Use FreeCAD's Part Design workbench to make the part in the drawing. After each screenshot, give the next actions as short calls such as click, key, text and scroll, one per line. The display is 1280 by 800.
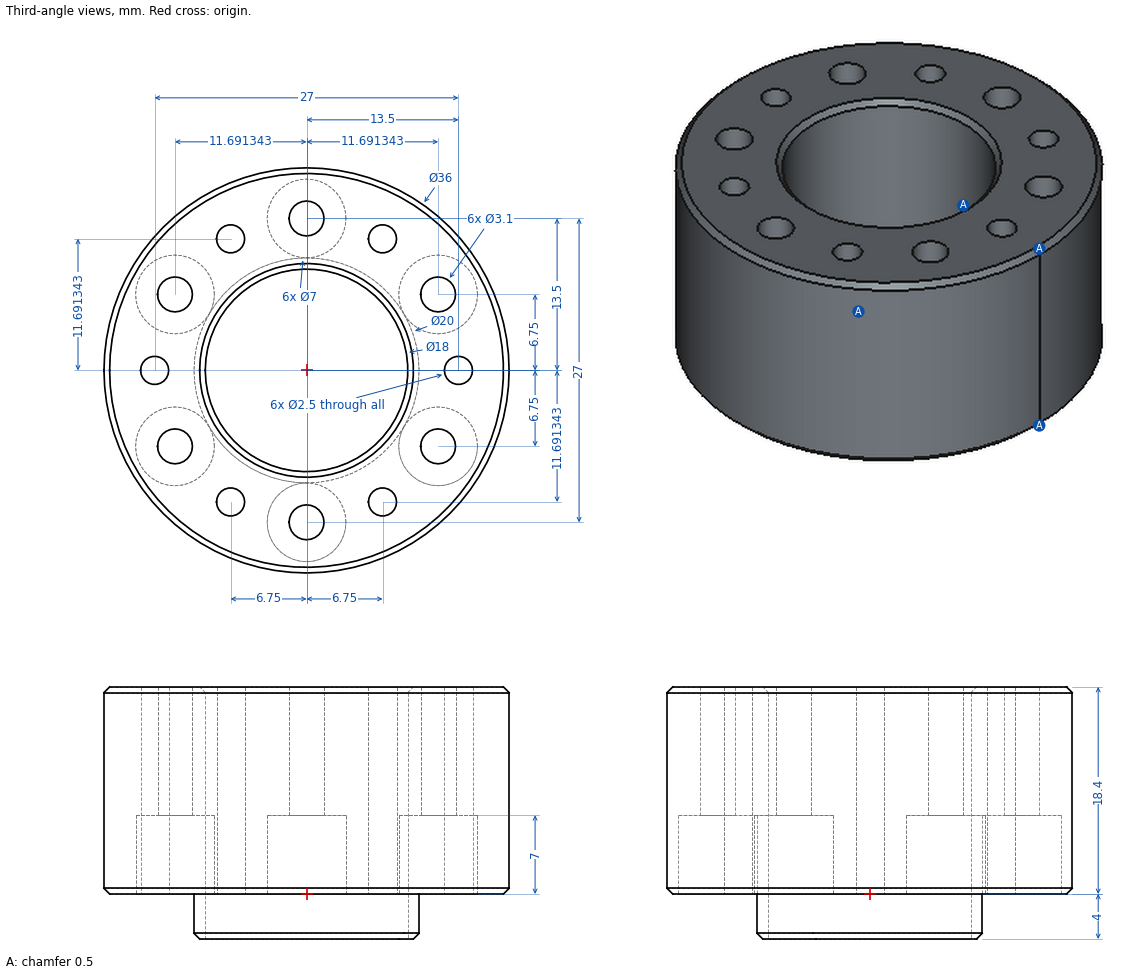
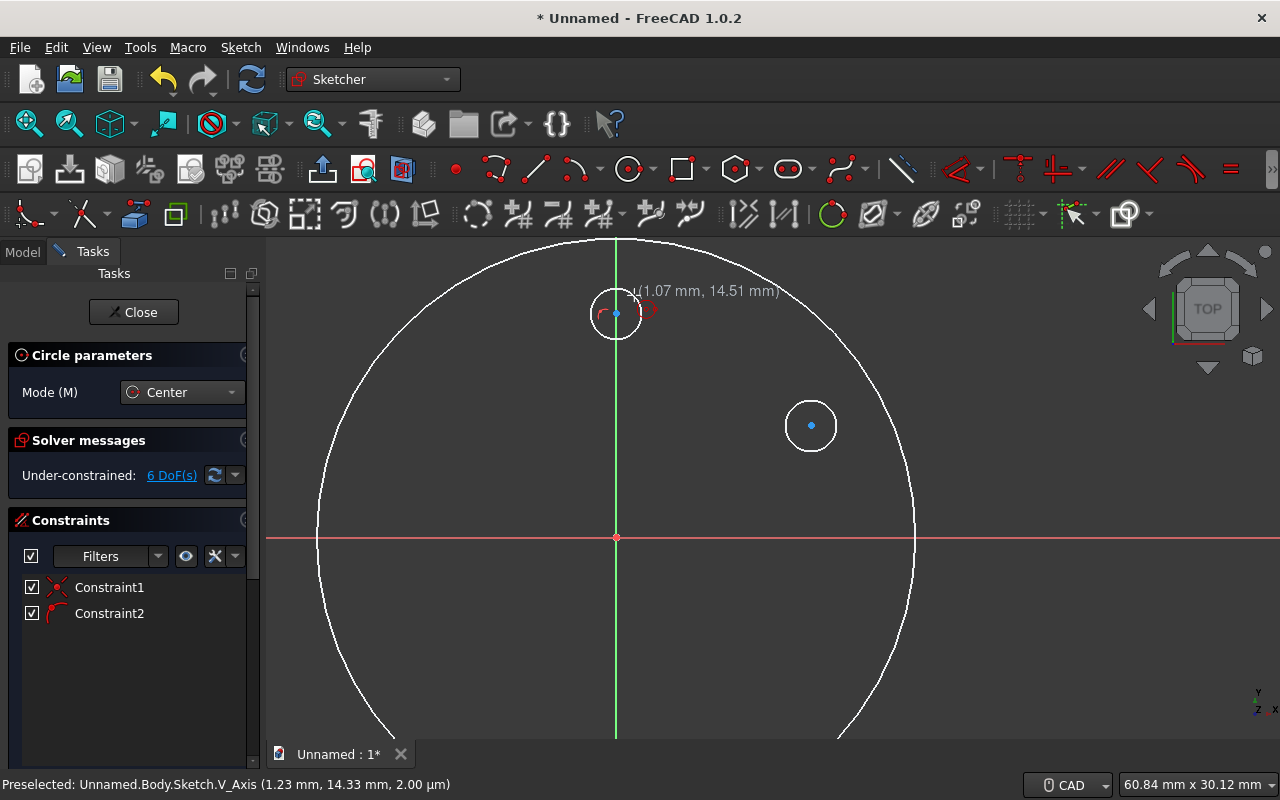
click(616, 538)
click(722, 432)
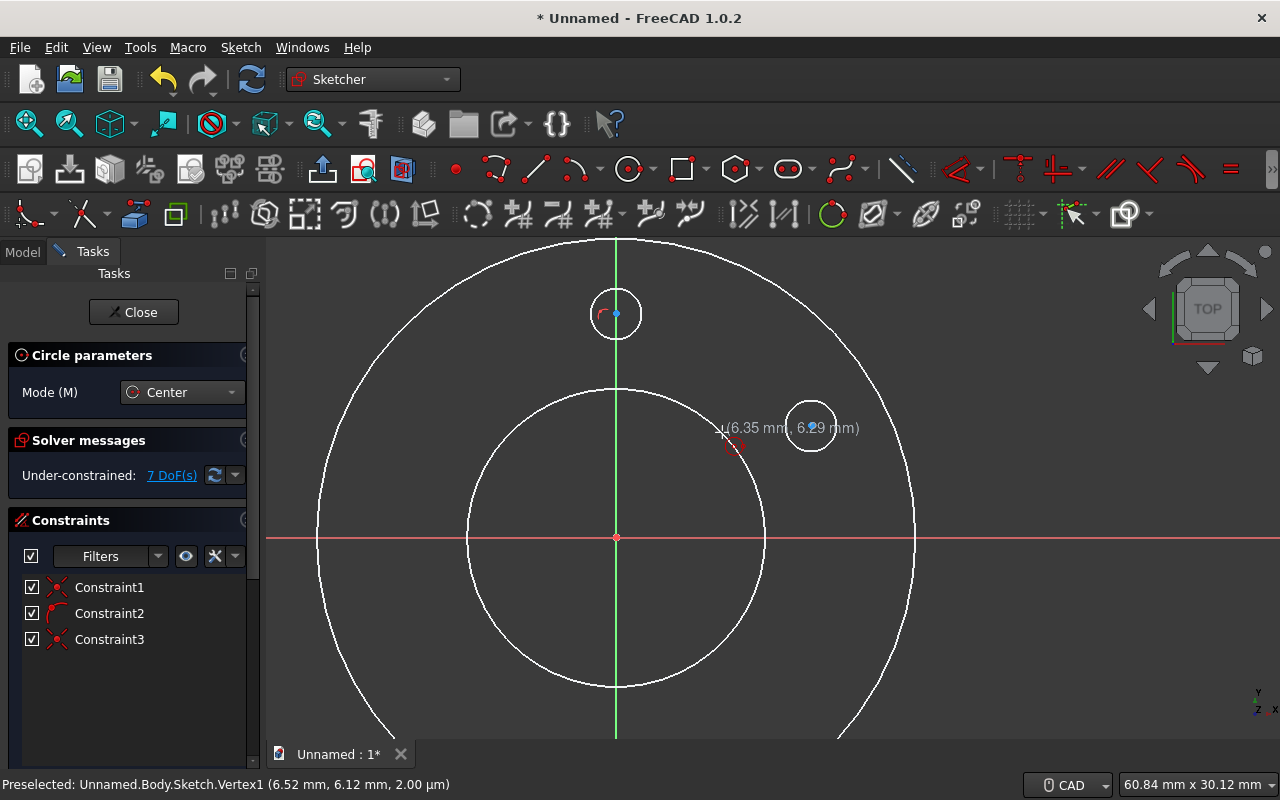
click(421, 425)
click(440, 407)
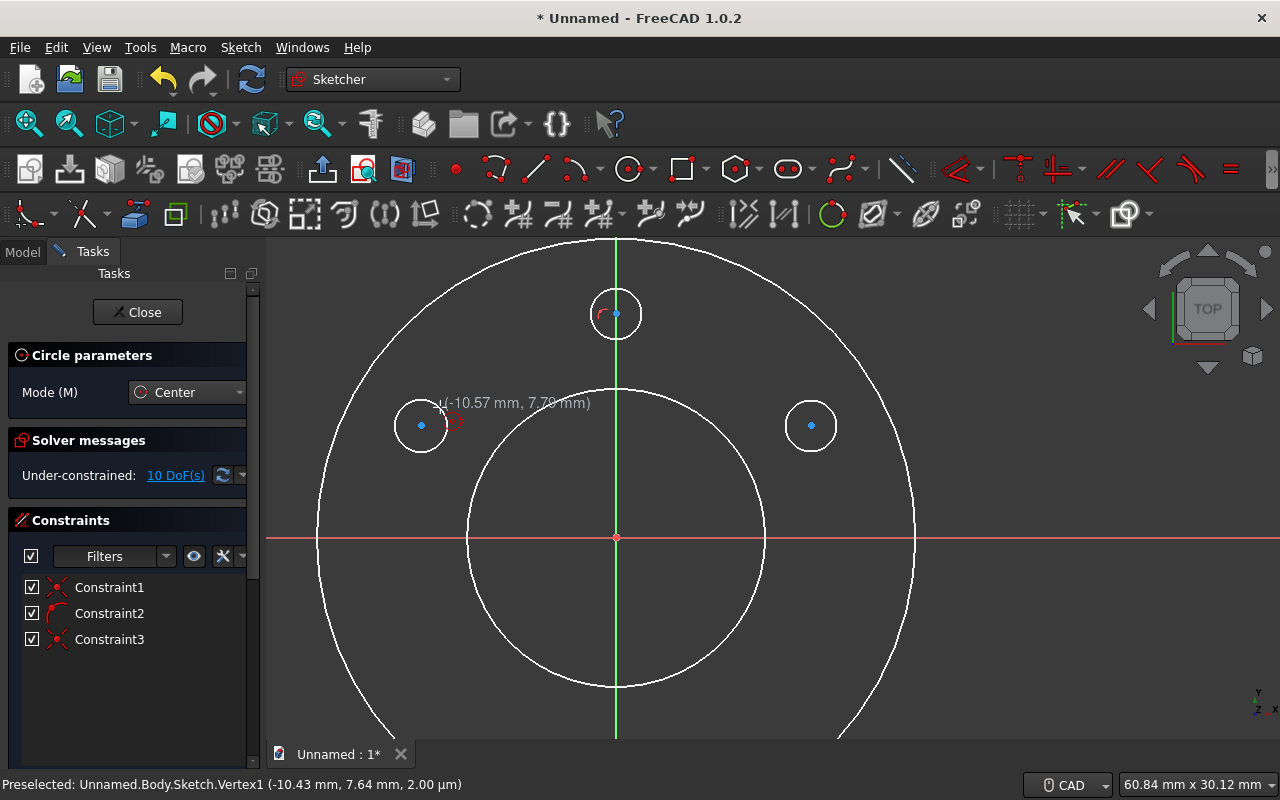
click(811, 650)
click(829, 632)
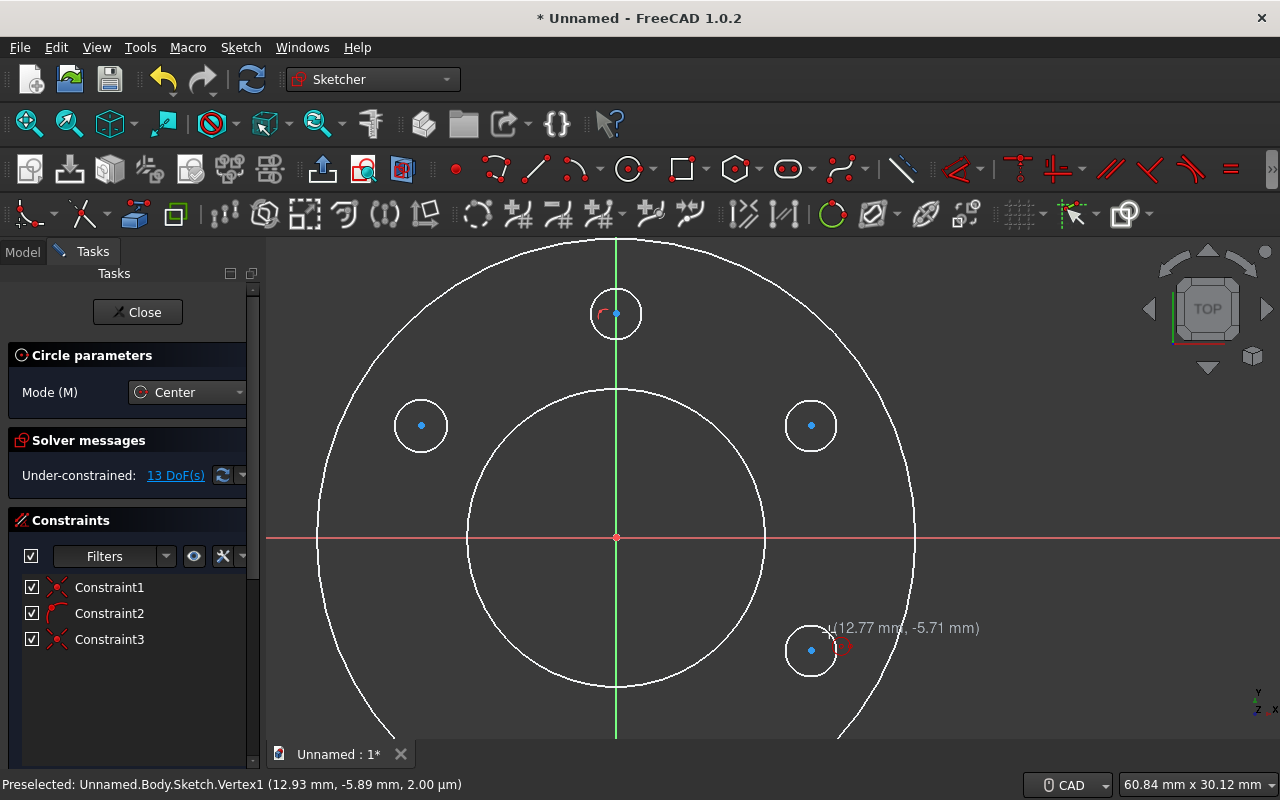
scroll(812, 427, down, 3)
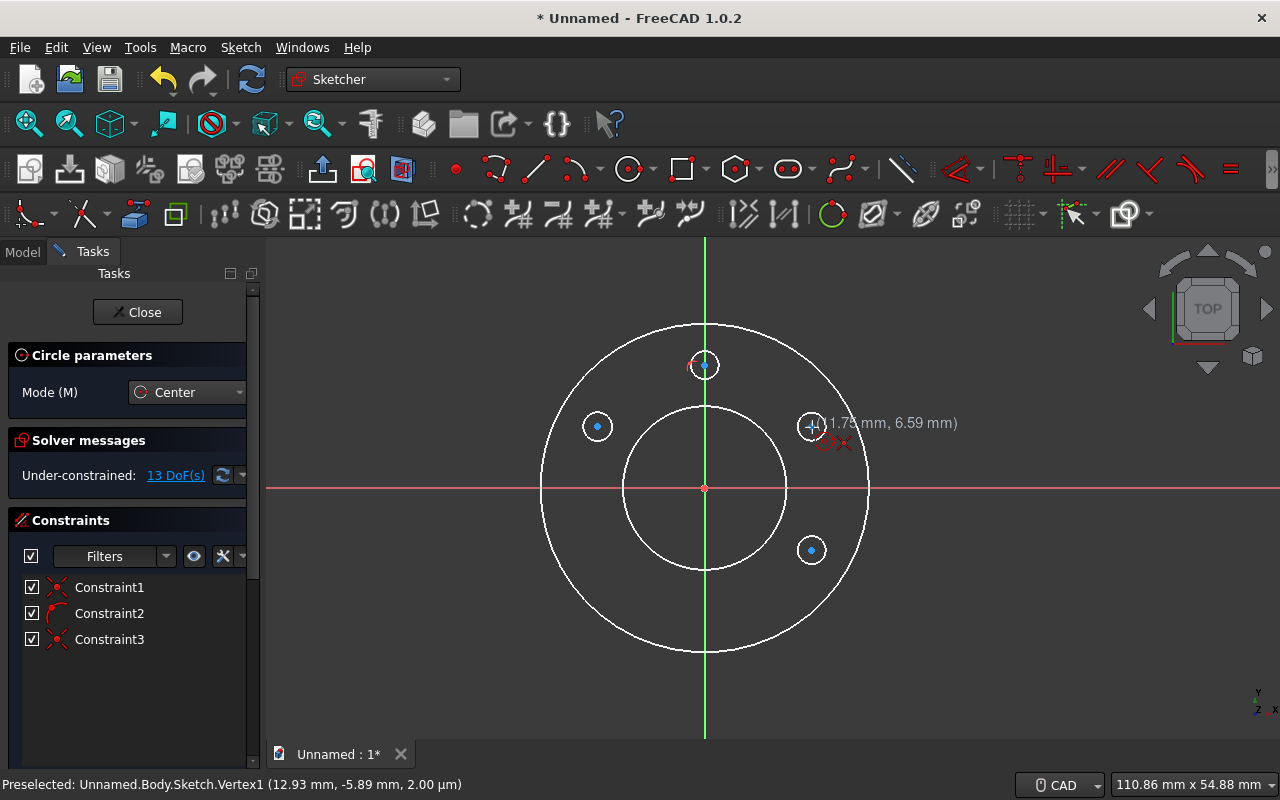
scroll(705, 612, up, 3)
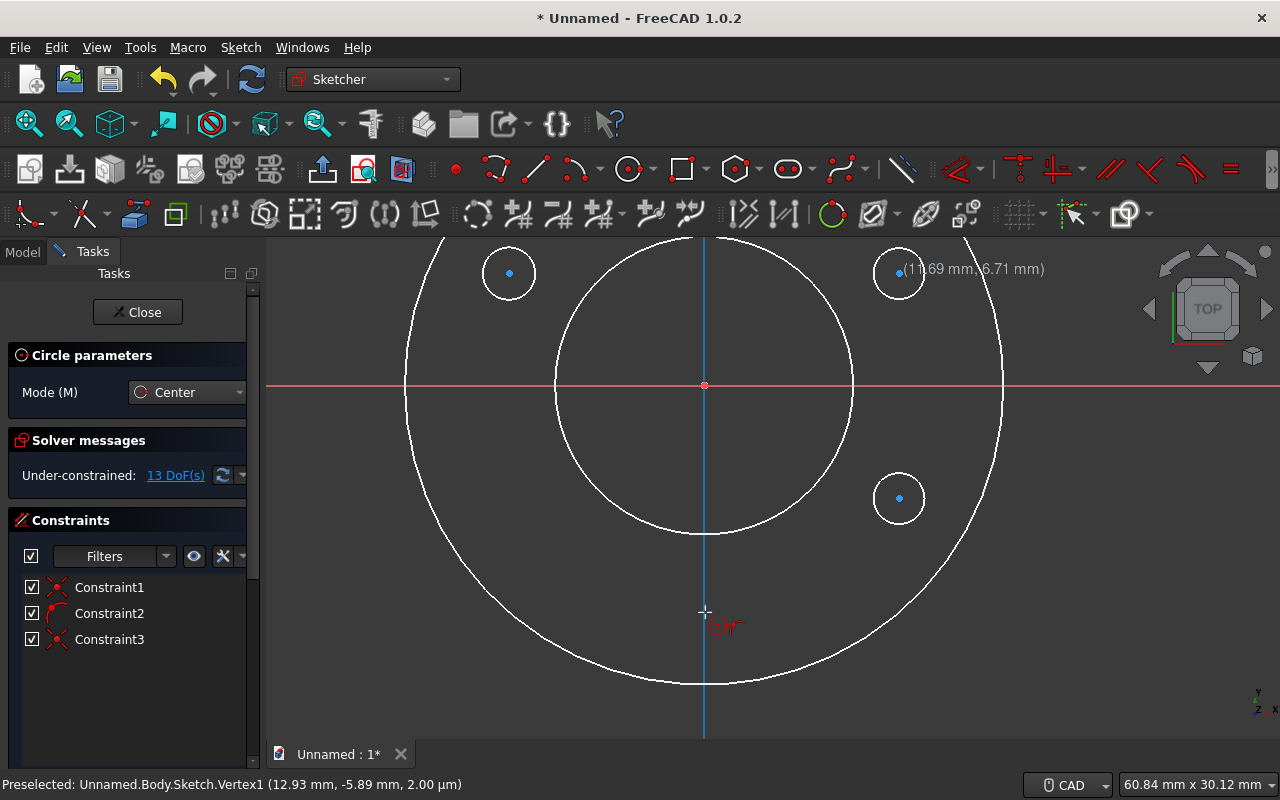
click(704, 611)
click(722, 592)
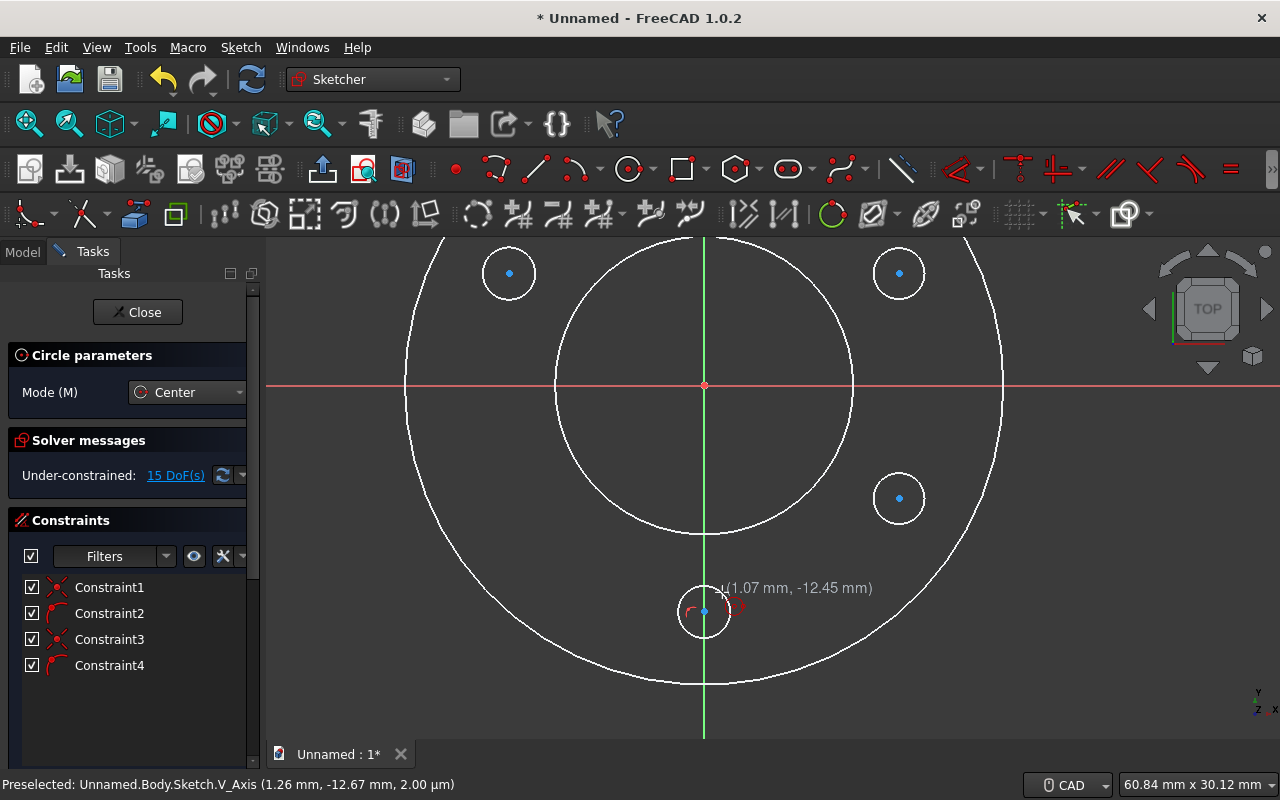
click(509, 498)
click(528, 480)
key(Escape)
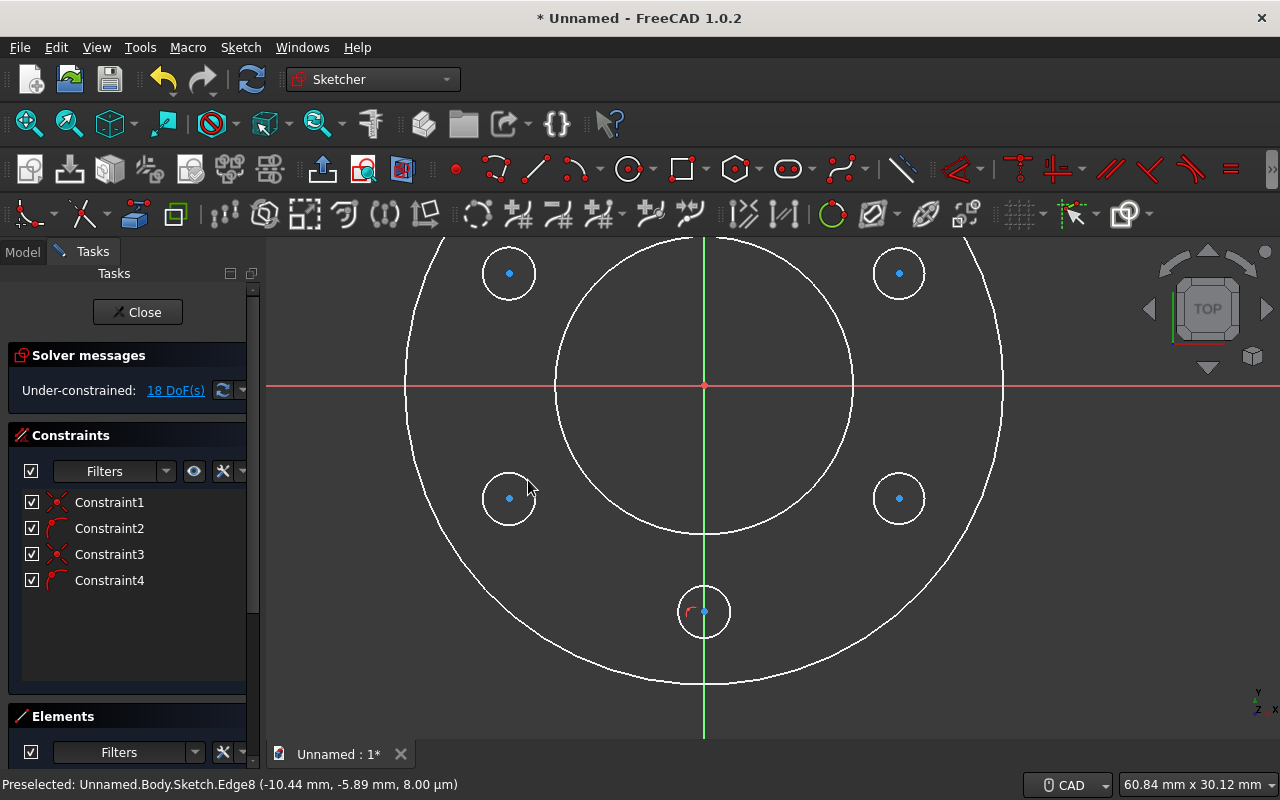
click(881, 292)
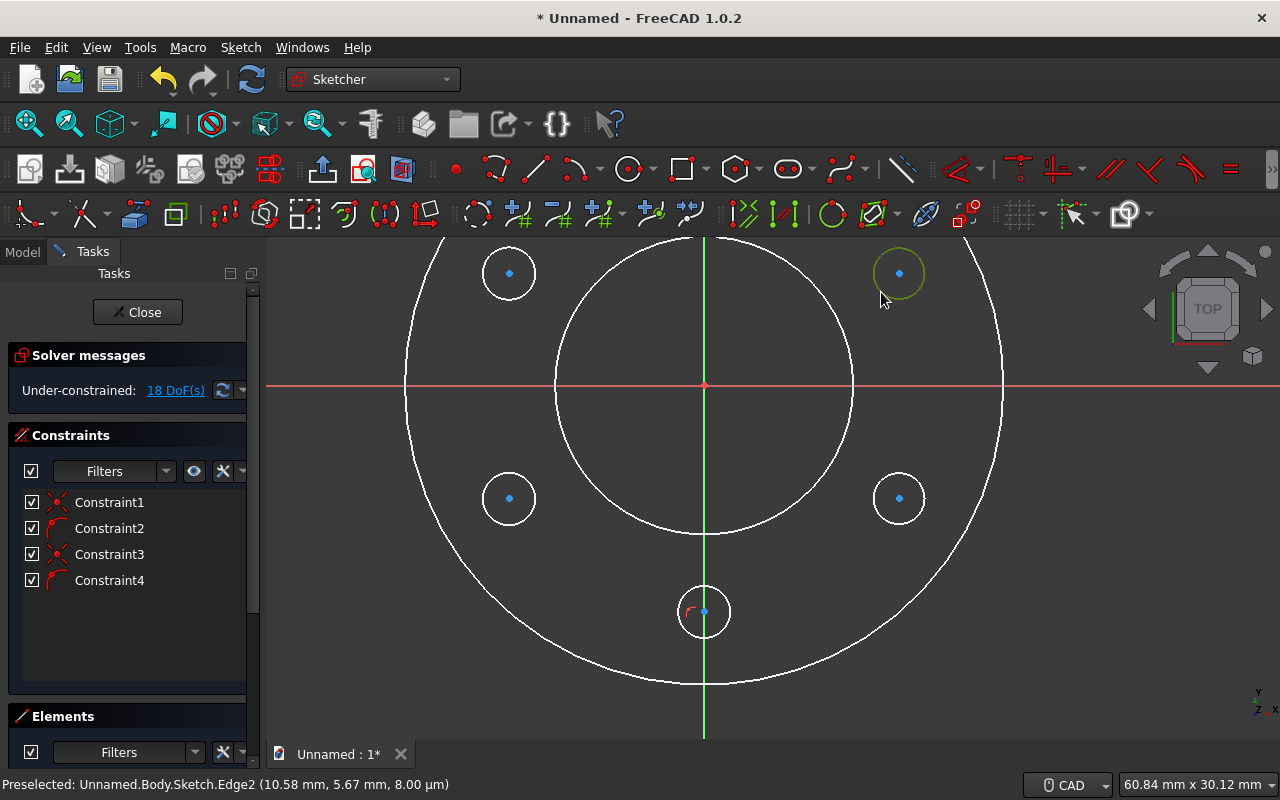
scroll(705, 613, down, 3)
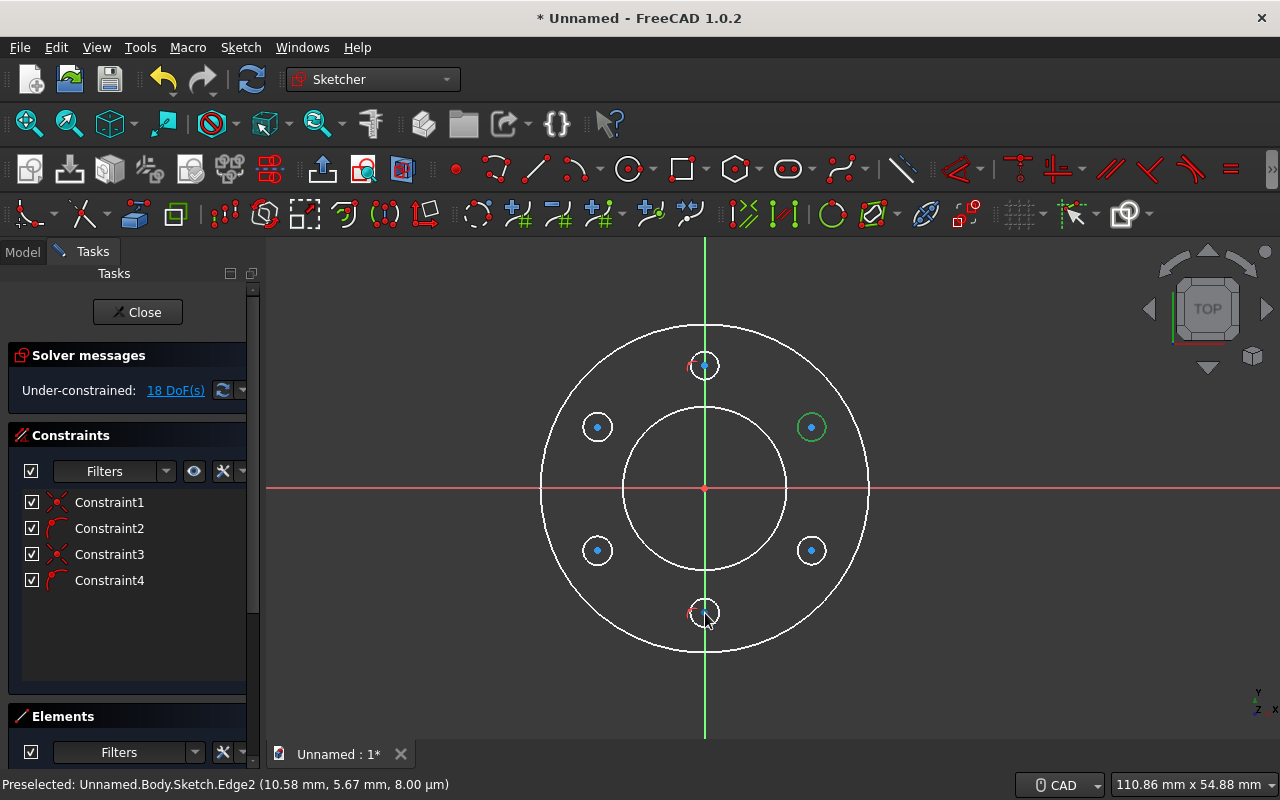
scroll(715, 356, up, 2)